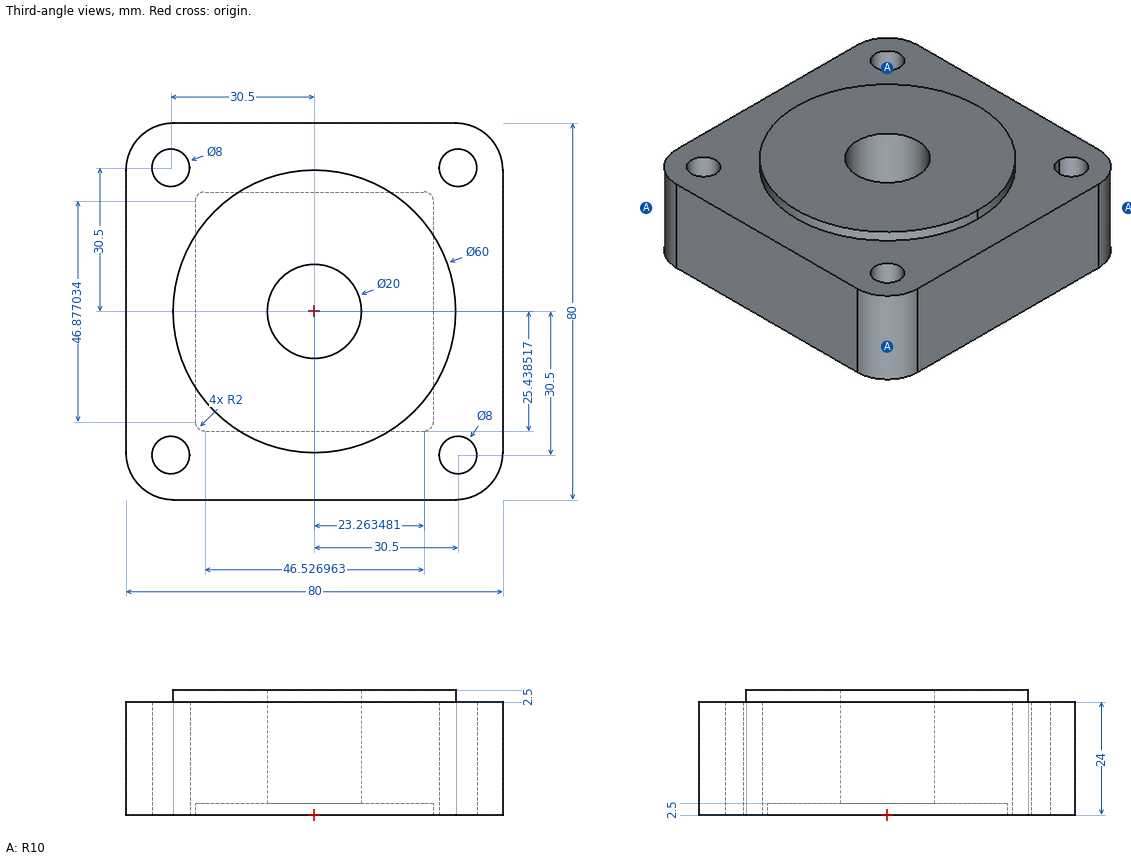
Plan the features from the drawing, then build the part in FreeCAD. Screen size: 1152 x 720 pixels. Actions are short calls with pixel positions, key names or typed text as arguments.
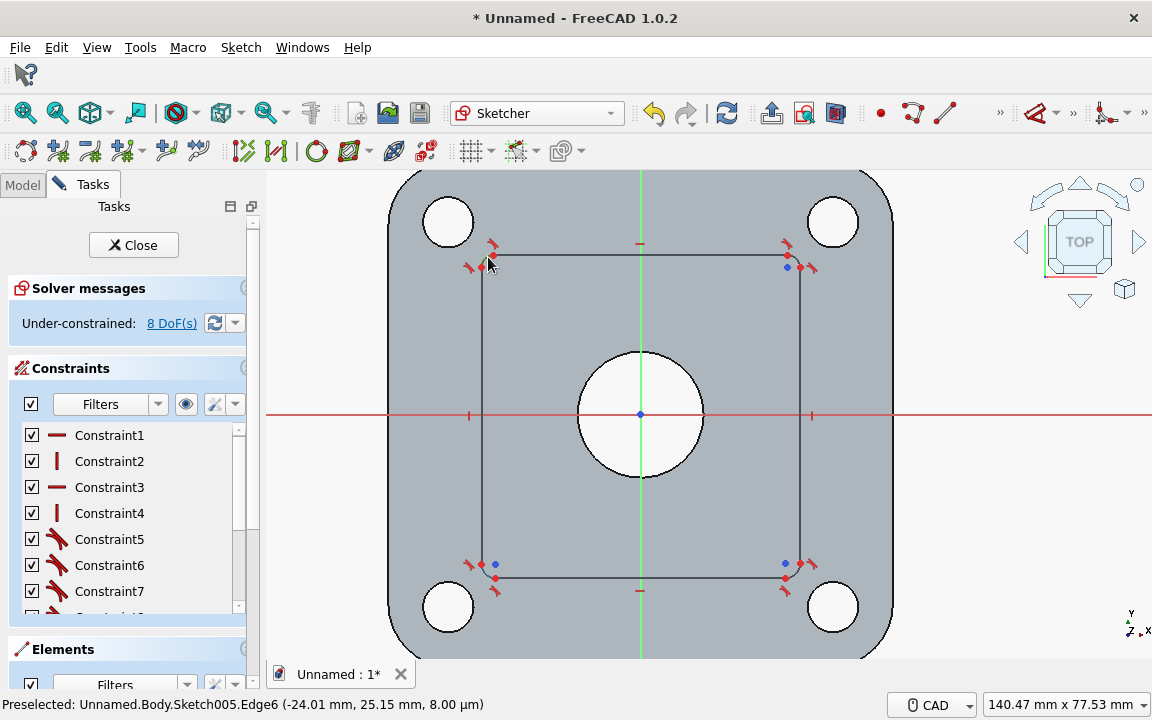
scroll(799, 262, up, 5)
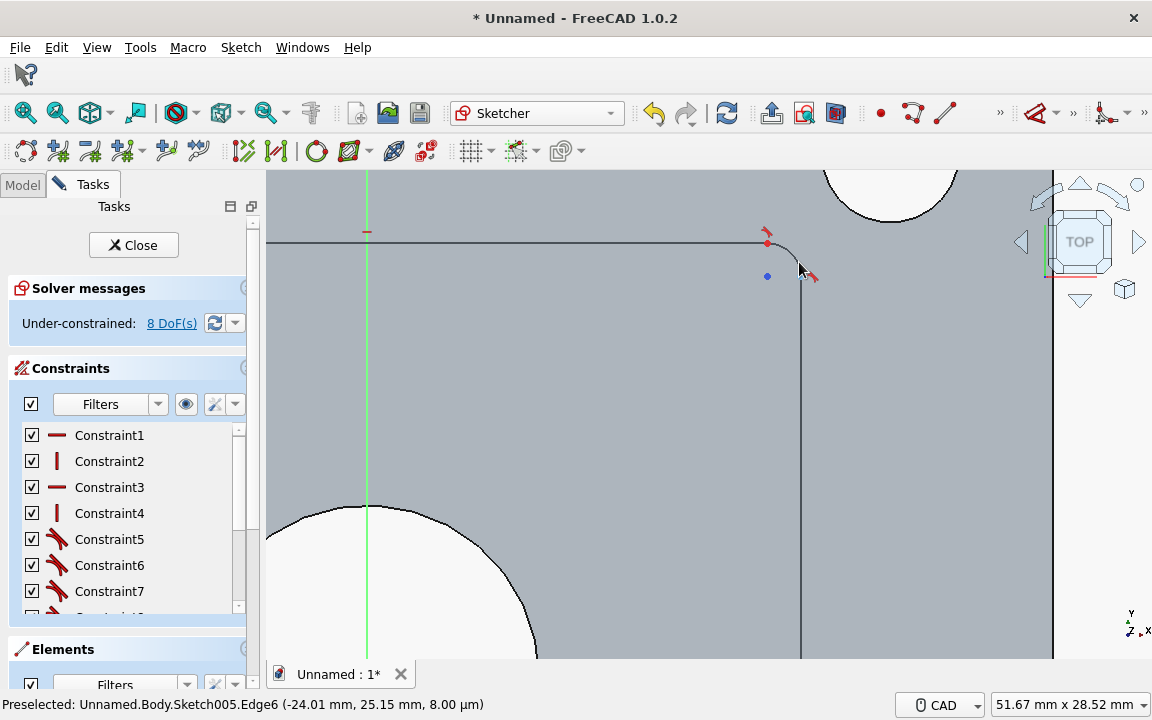
click(797, 262)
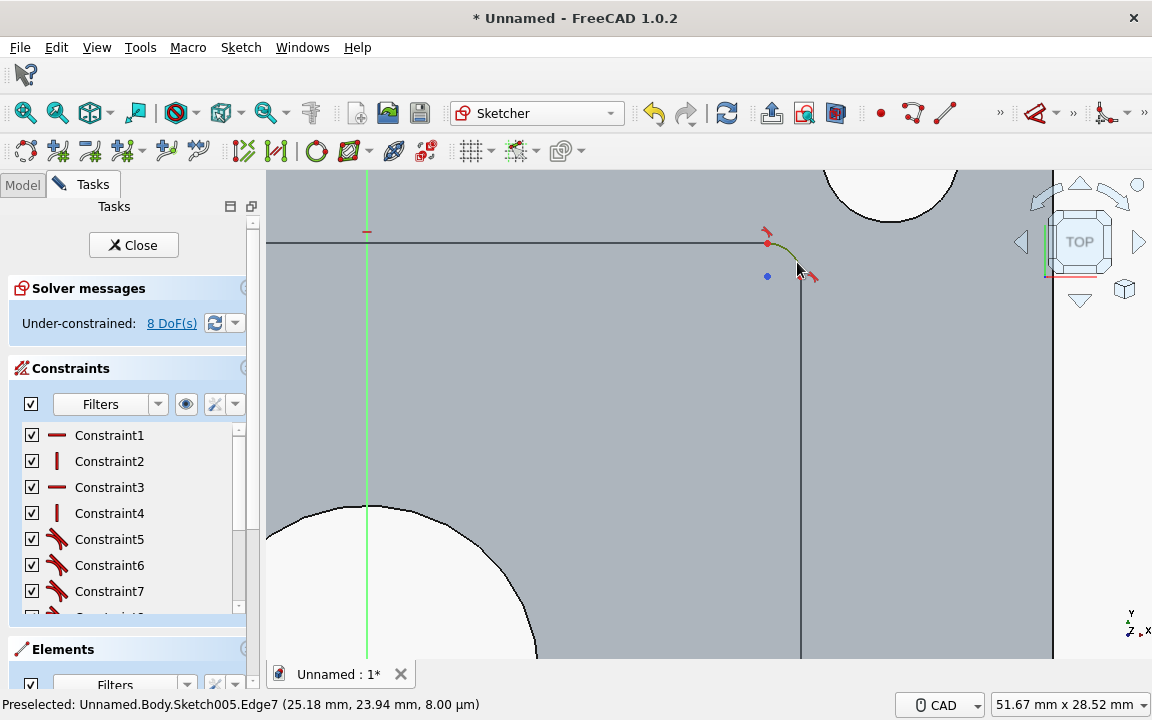
scroll(799, 262, down, 5)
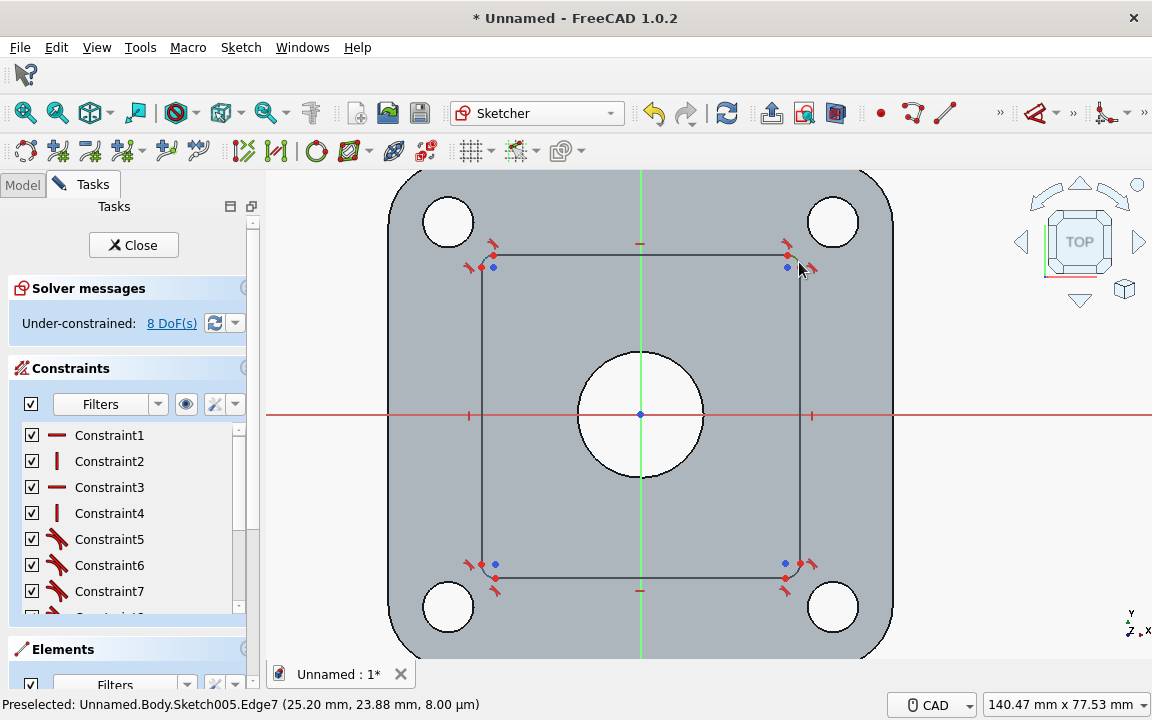
scroll(792, 577, up, 4)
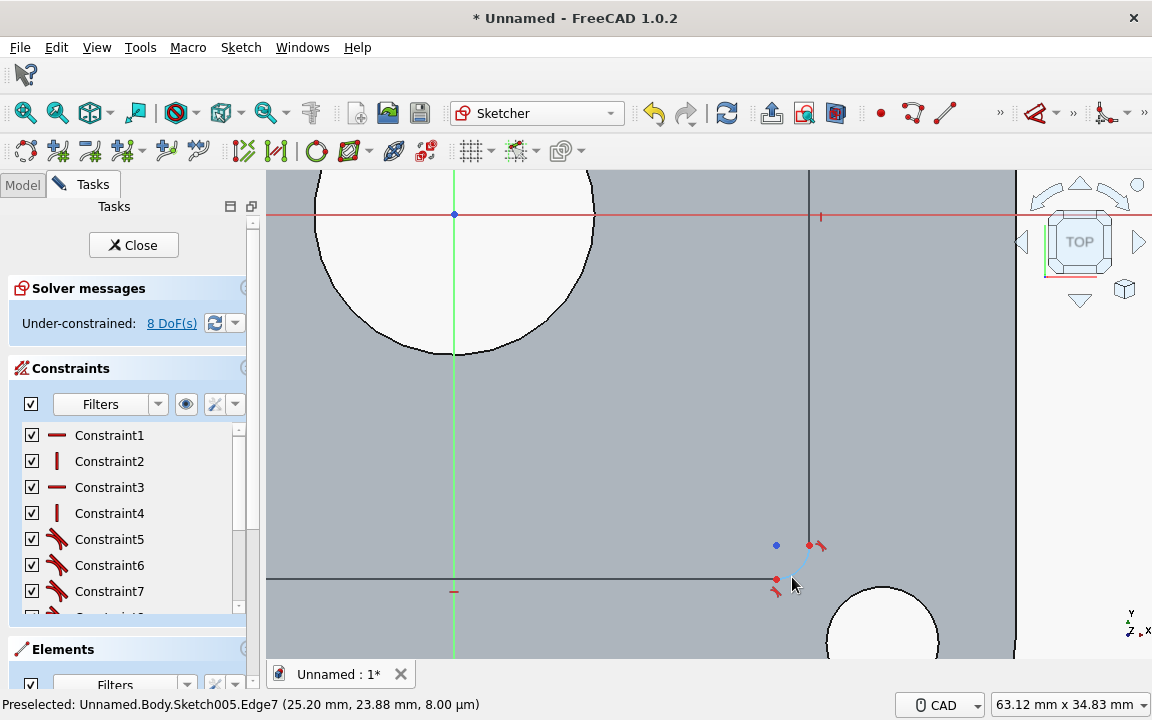
click(791, 575)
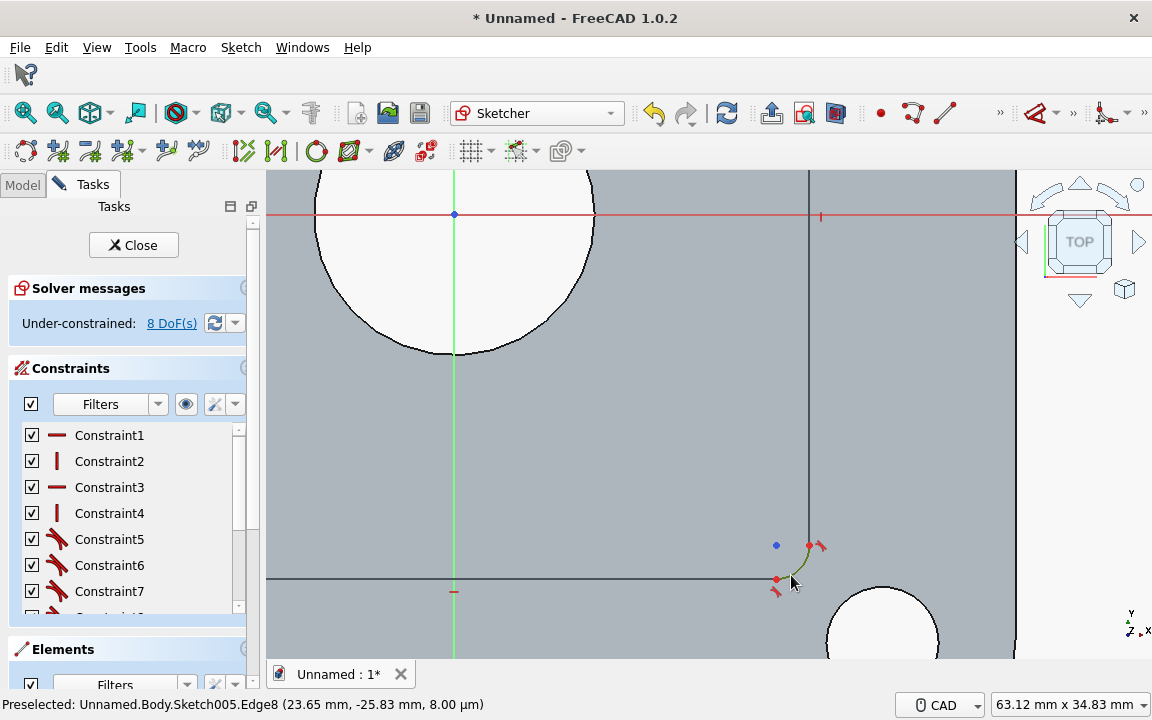
key(e)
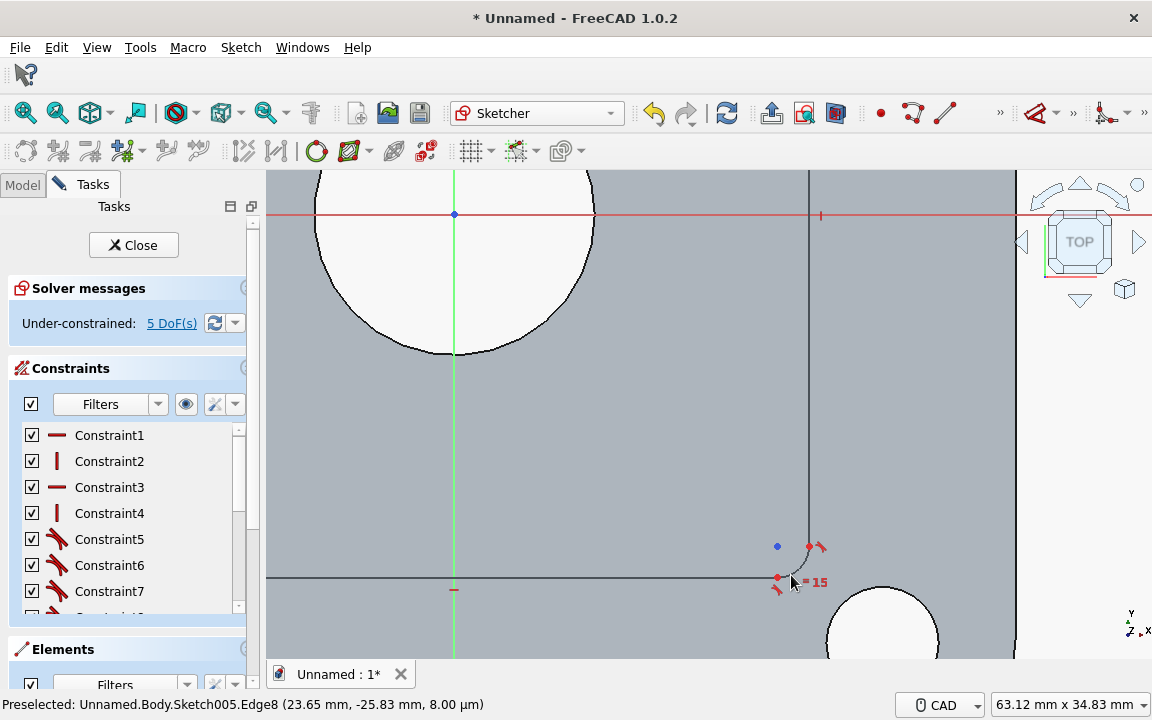
click(1036, 114)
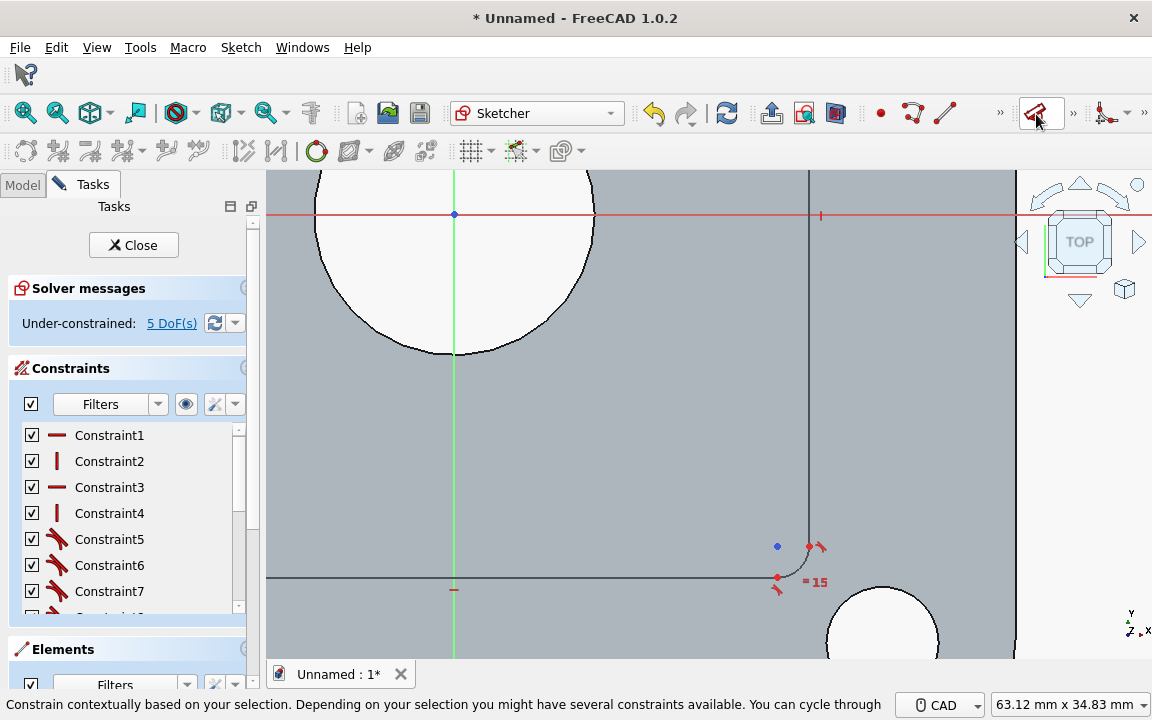
scroll(792, 577, down, 4)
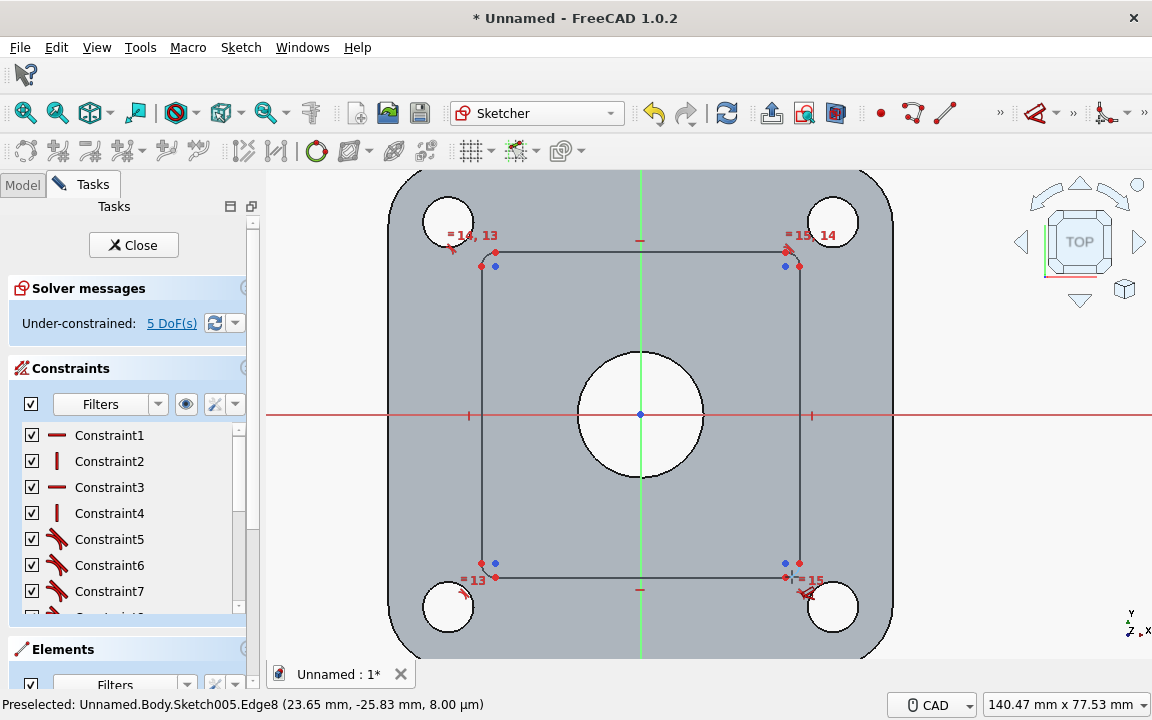
scroll(483, 570, up, 6)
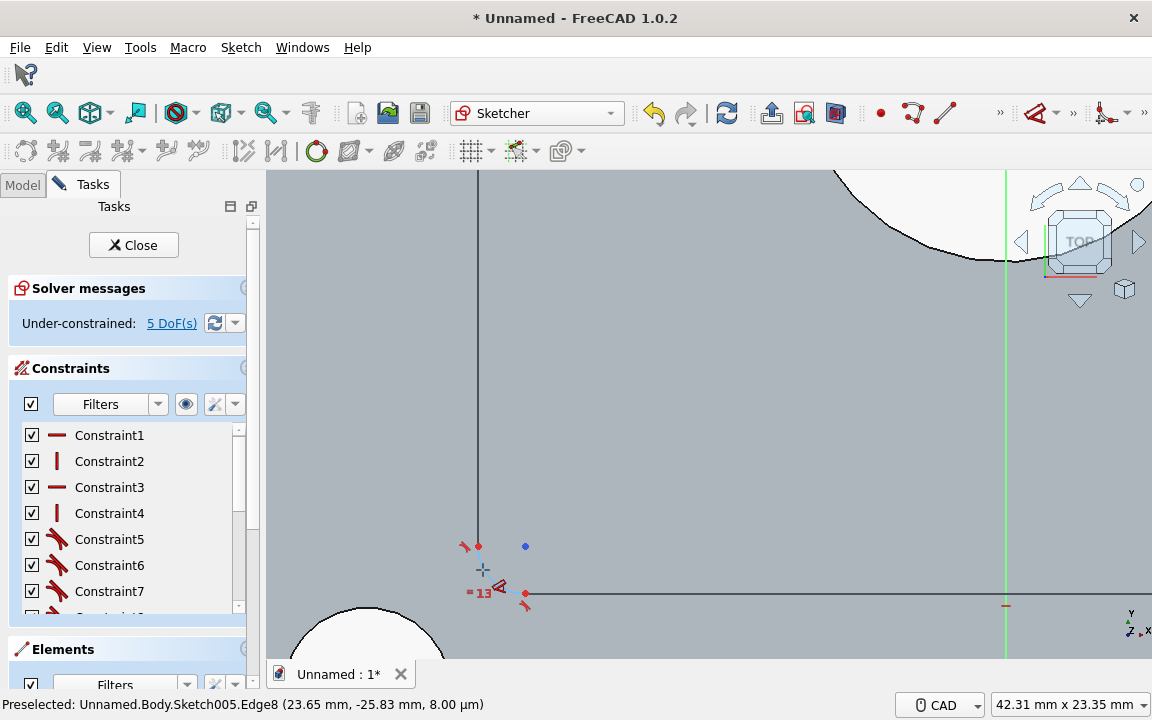
click(483, 568)
click(454, 582)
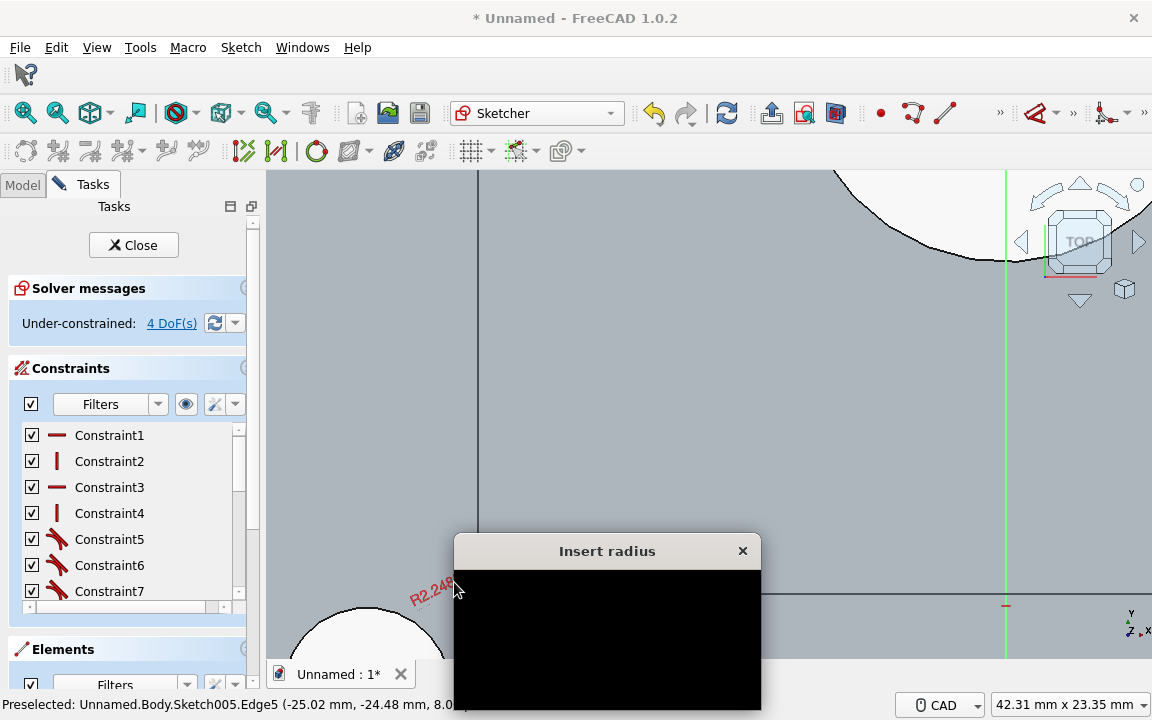
text(2)
key(Return)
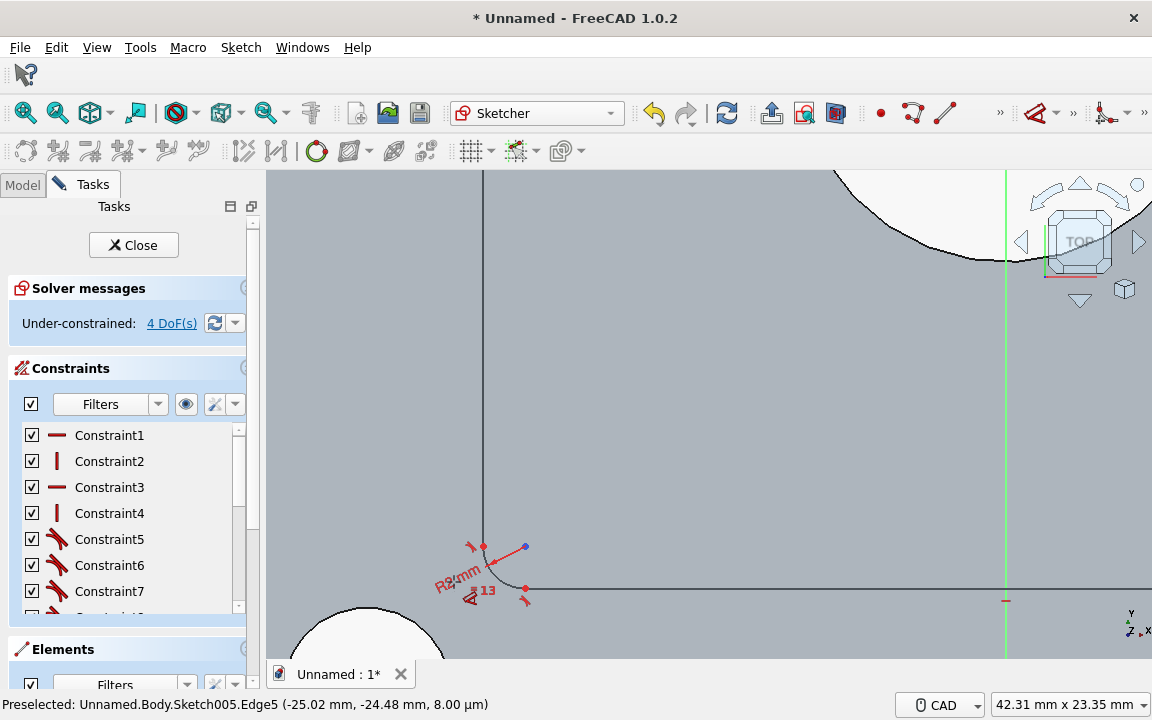
click(814, 589)
click(756, 623)